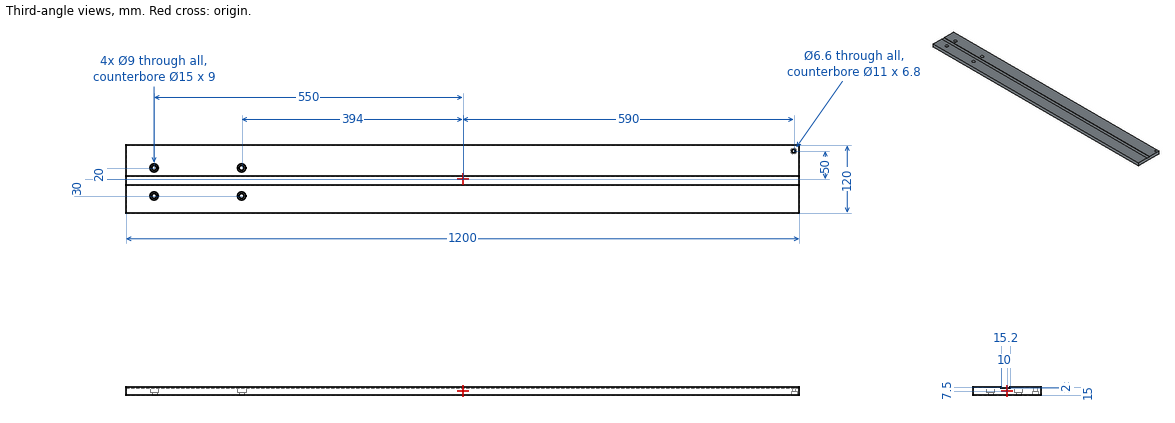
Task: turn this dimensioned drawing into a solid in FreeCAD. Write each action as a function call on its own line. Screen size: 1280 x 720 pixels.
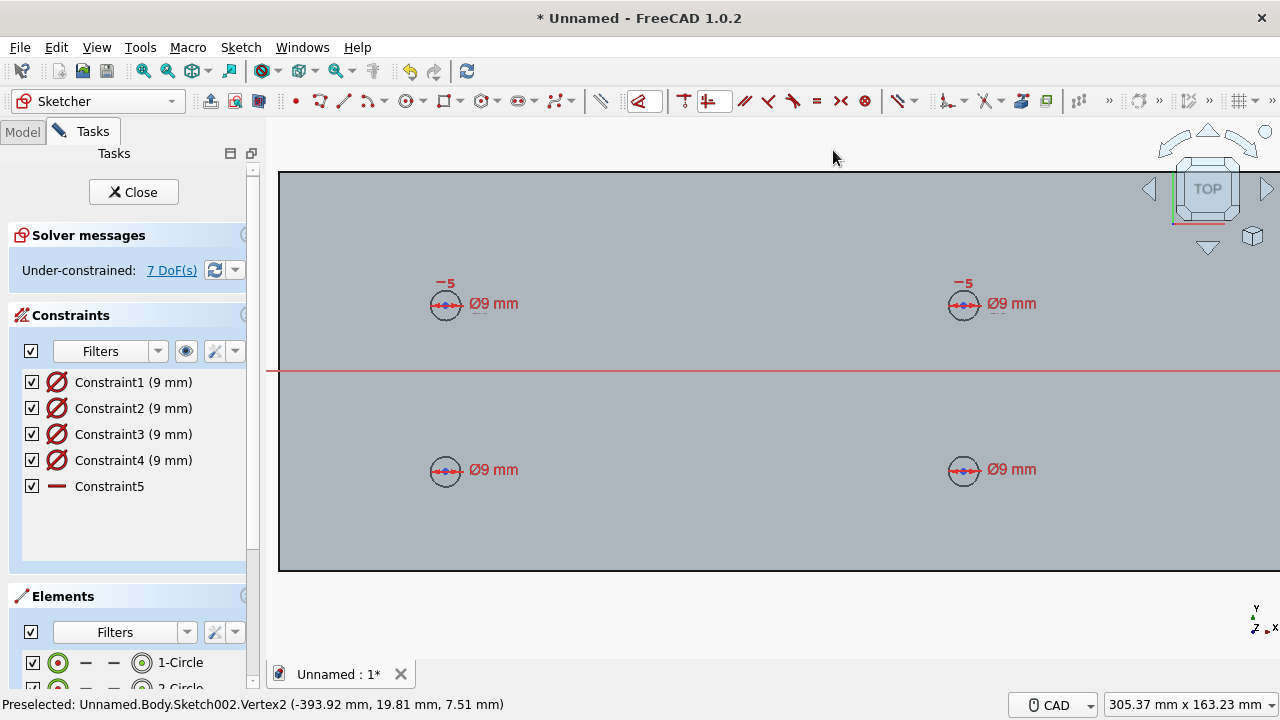
click(964, 306)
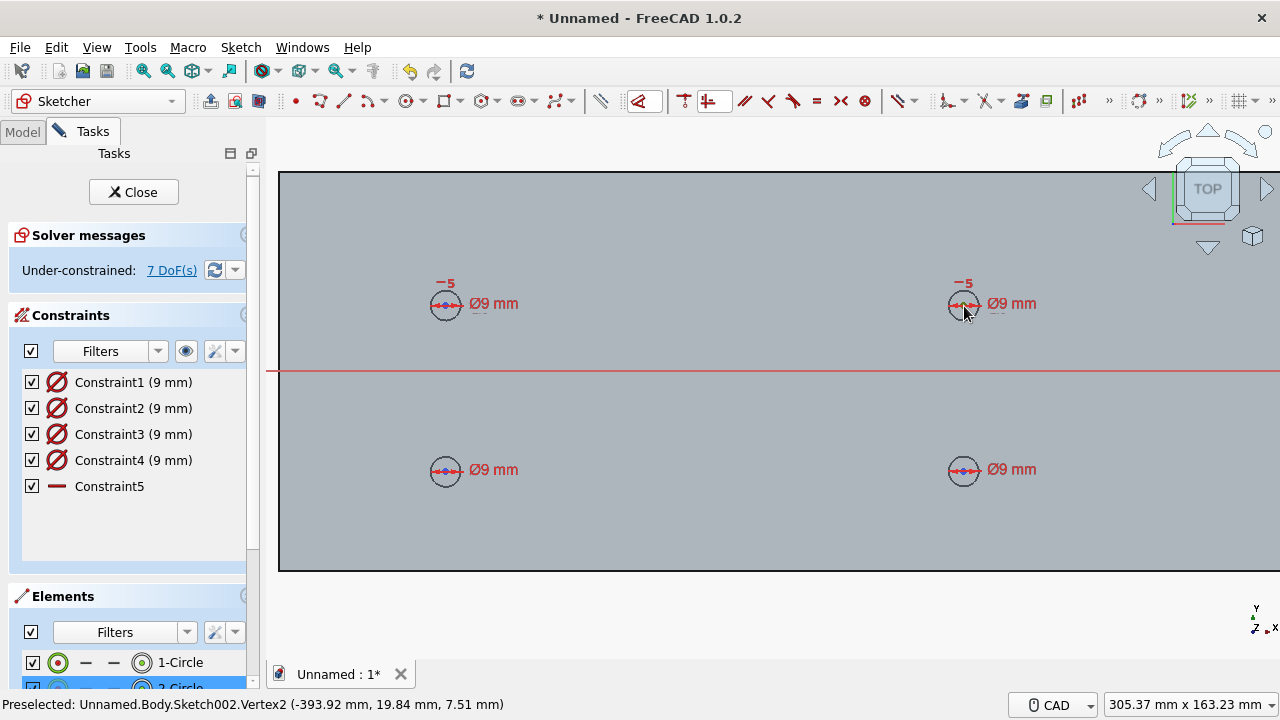
click(964, 471)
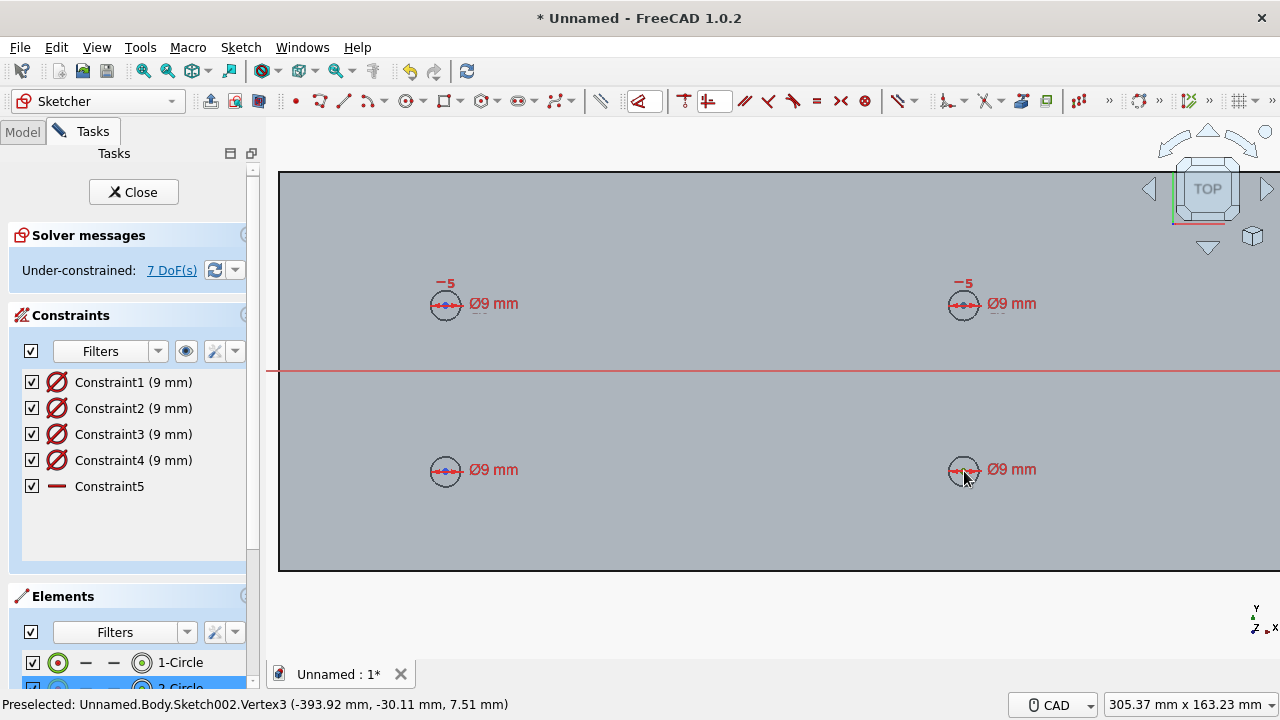
click(726, 102)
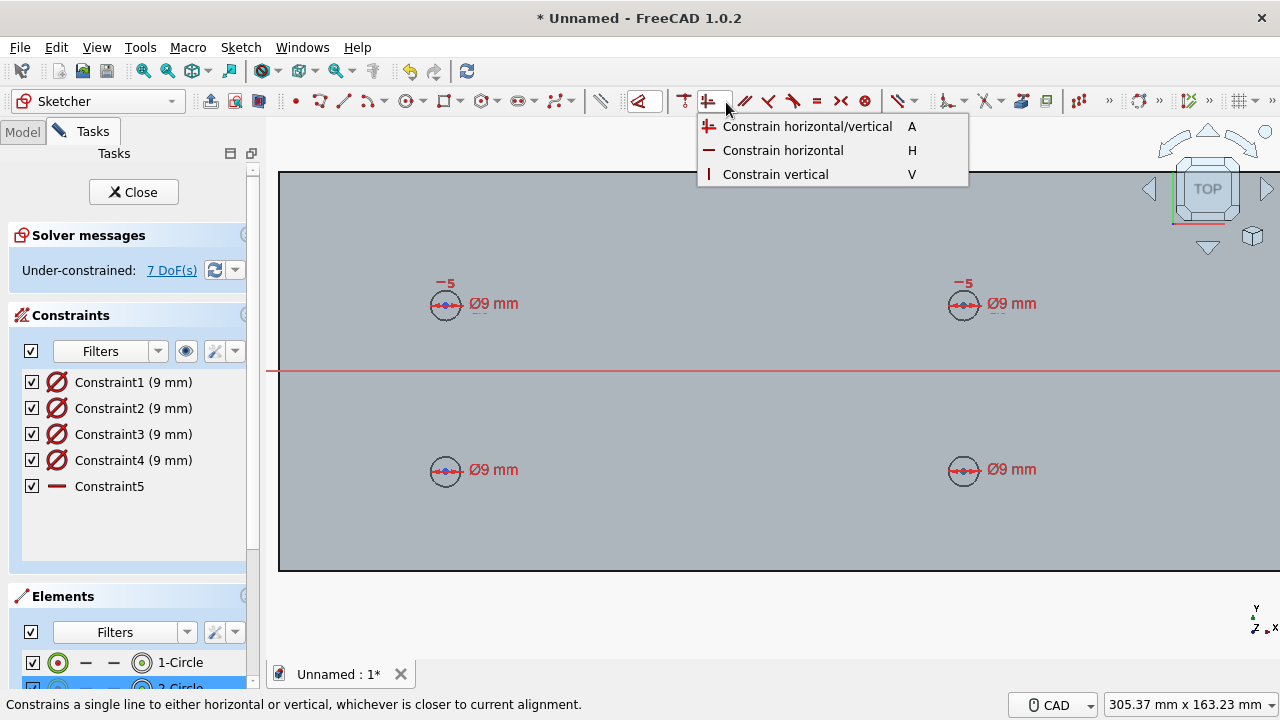
click(833, 174)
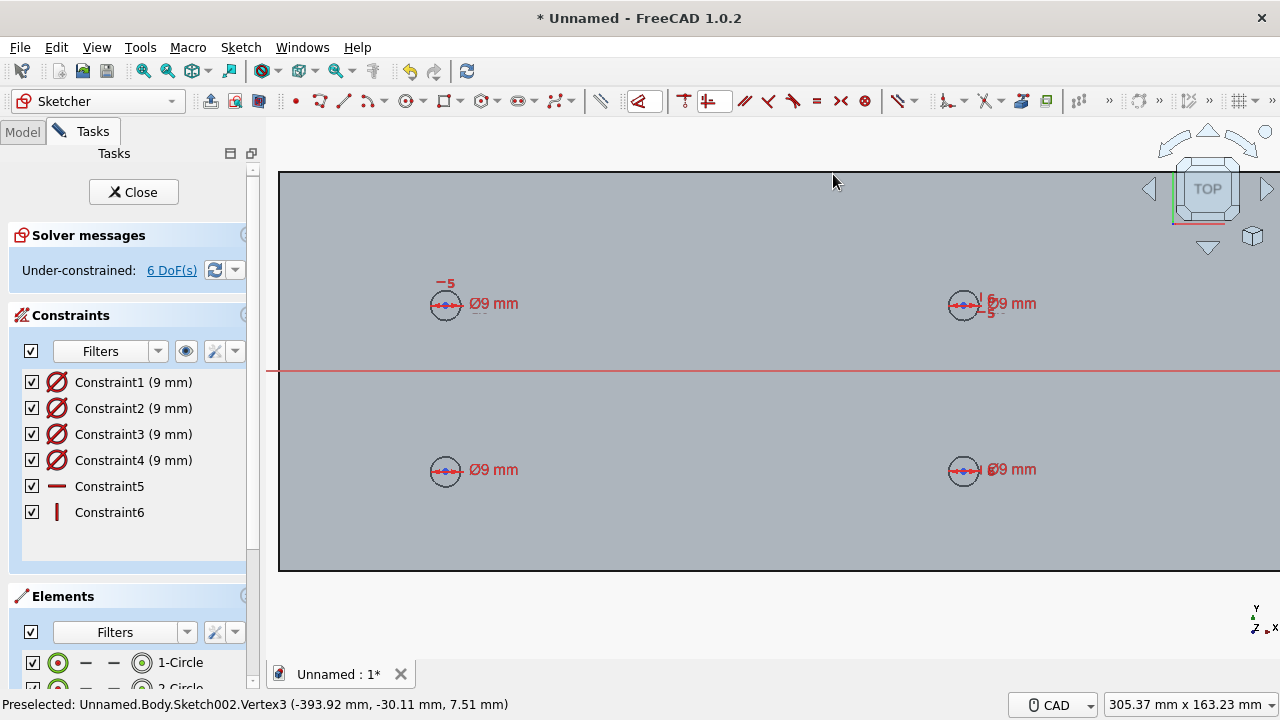
click(446, 306)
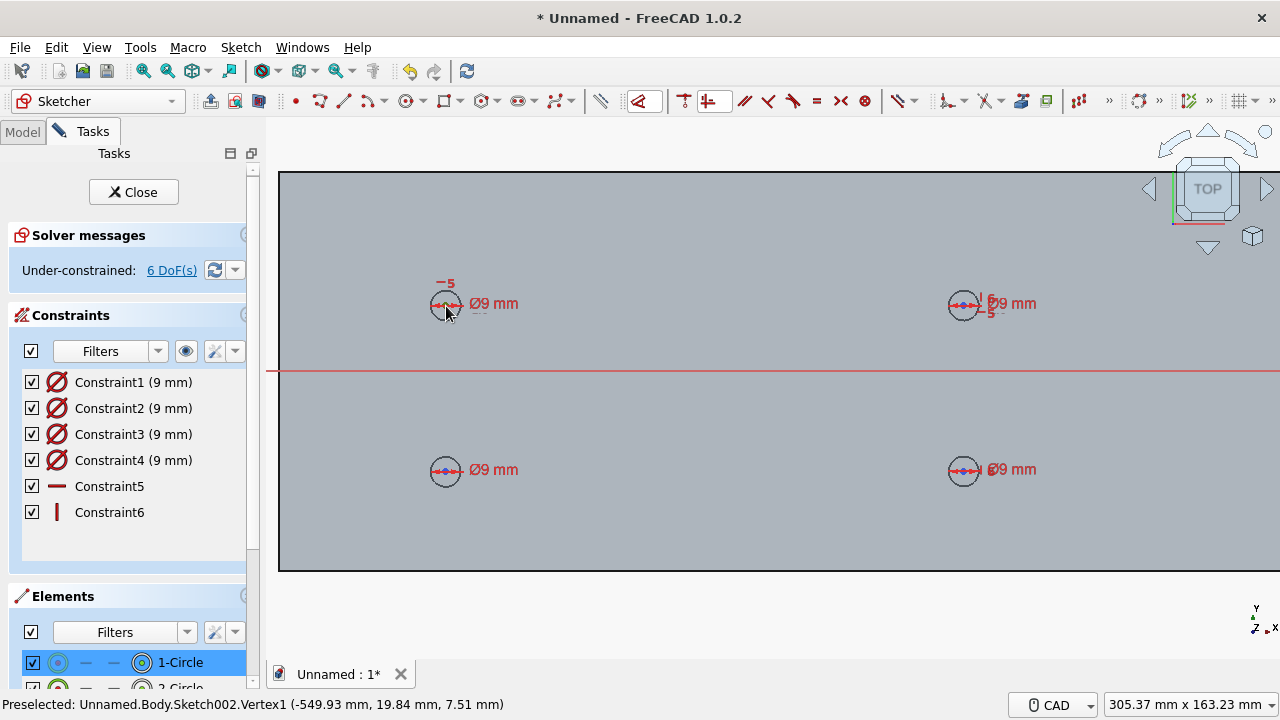
click(446, 472)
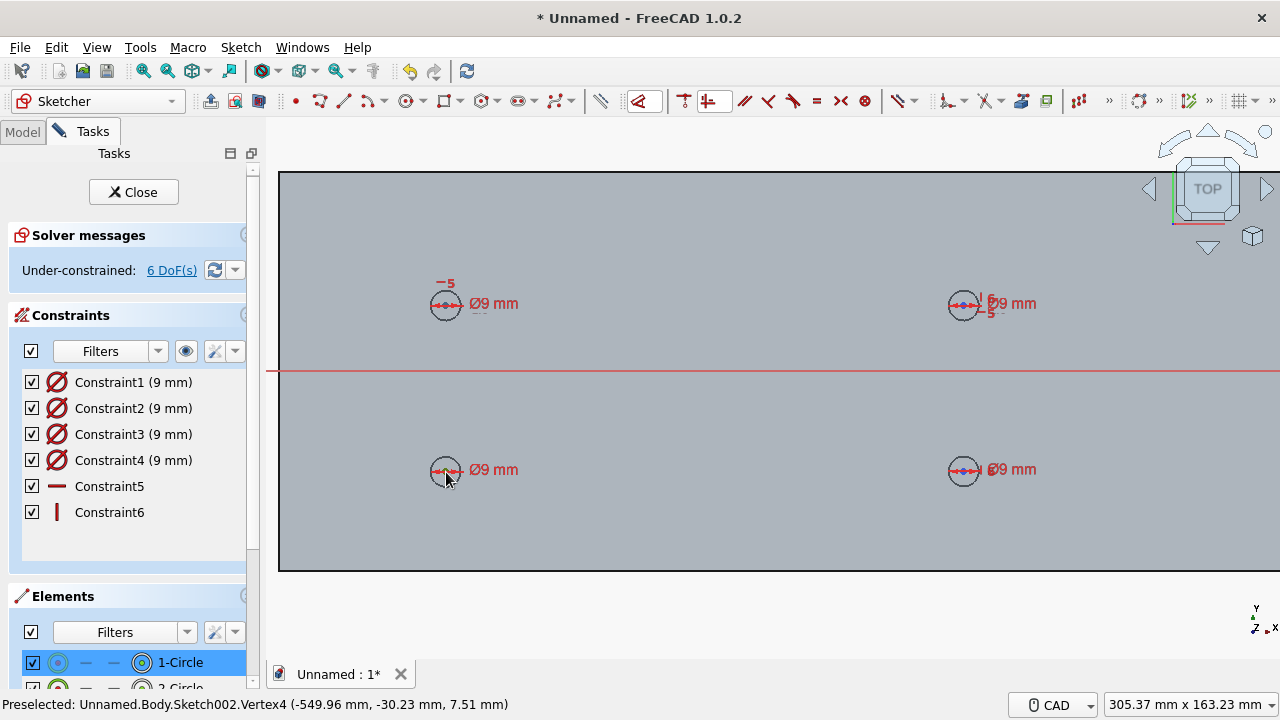
click(726, 102)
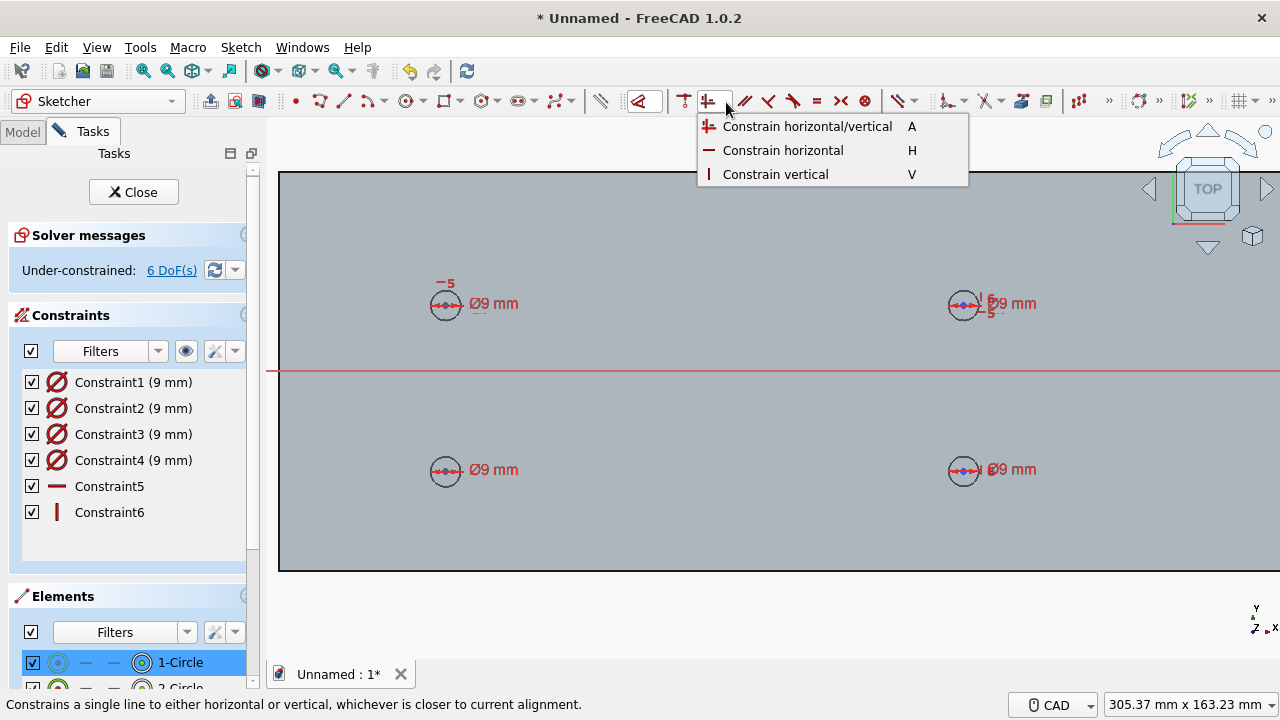
click(833, 174)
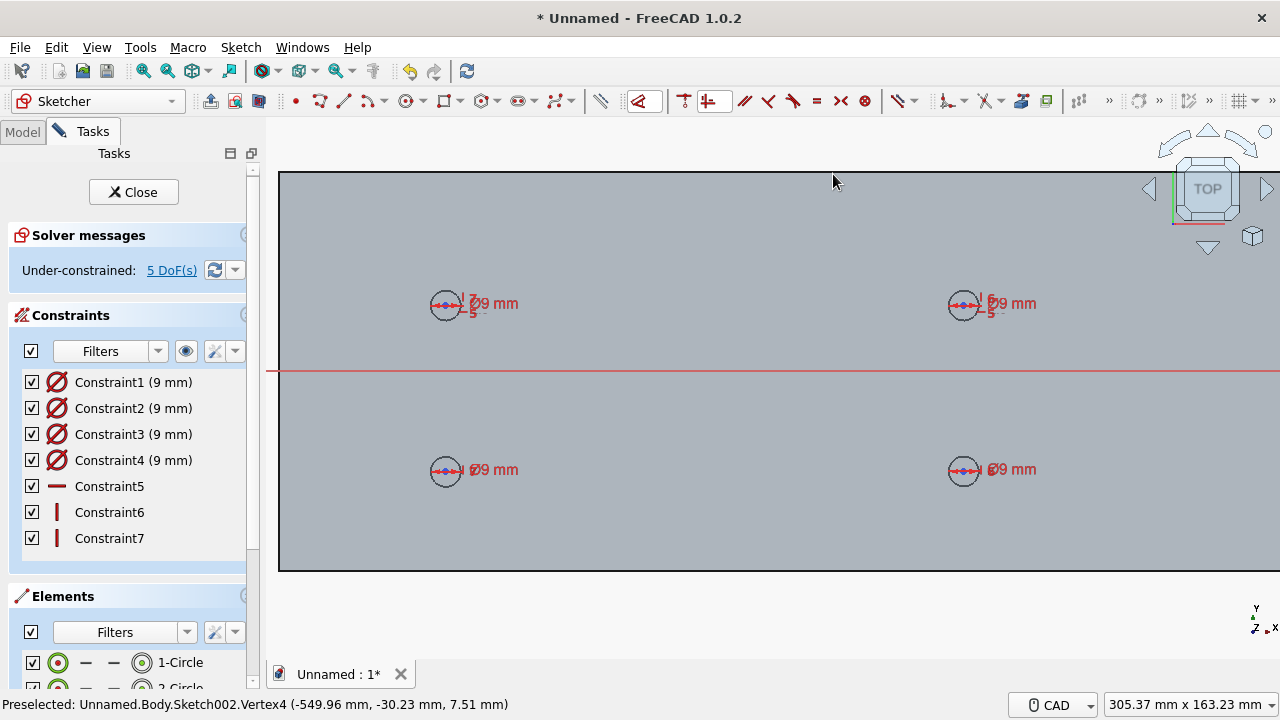
click(964, 471)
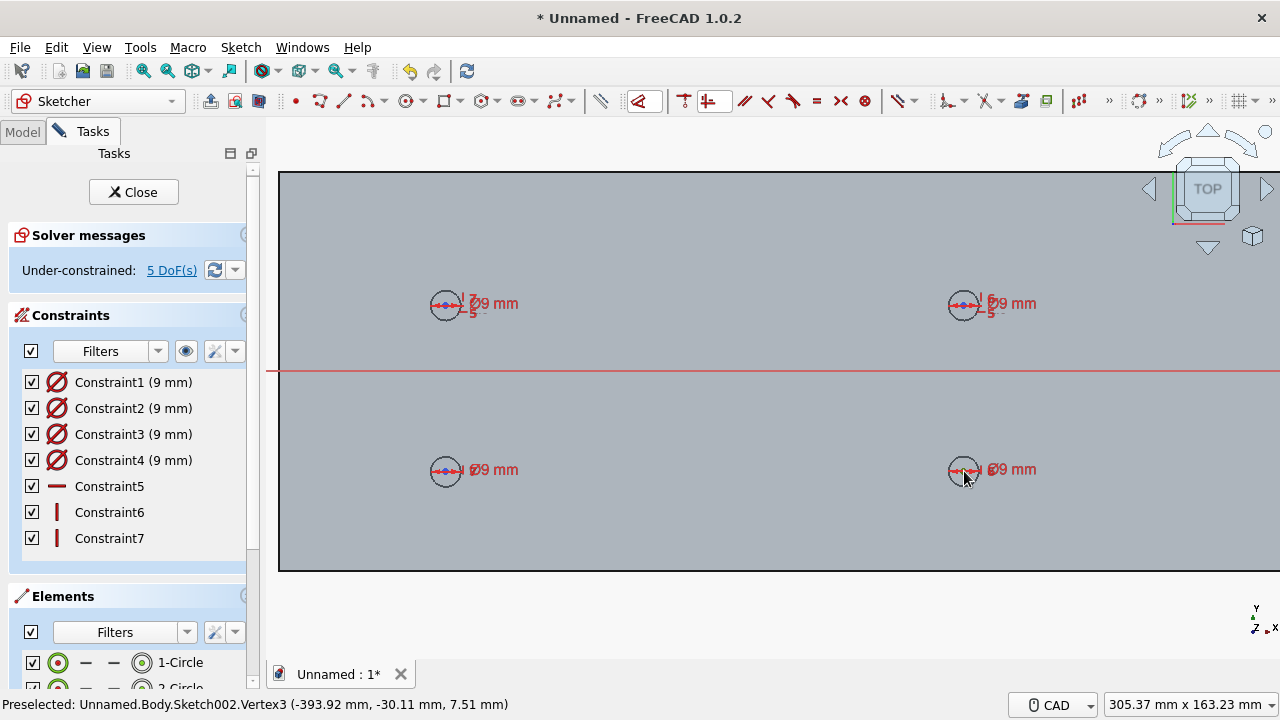
click(446, 472)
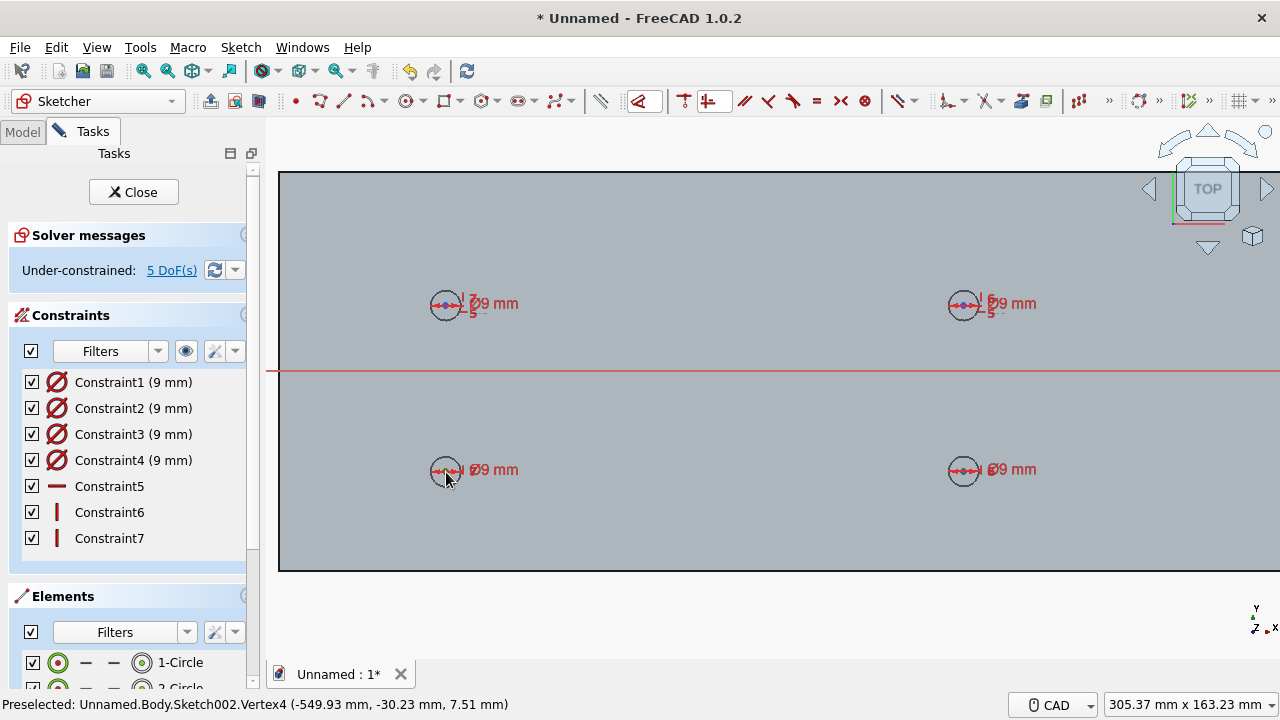
click(726, 102)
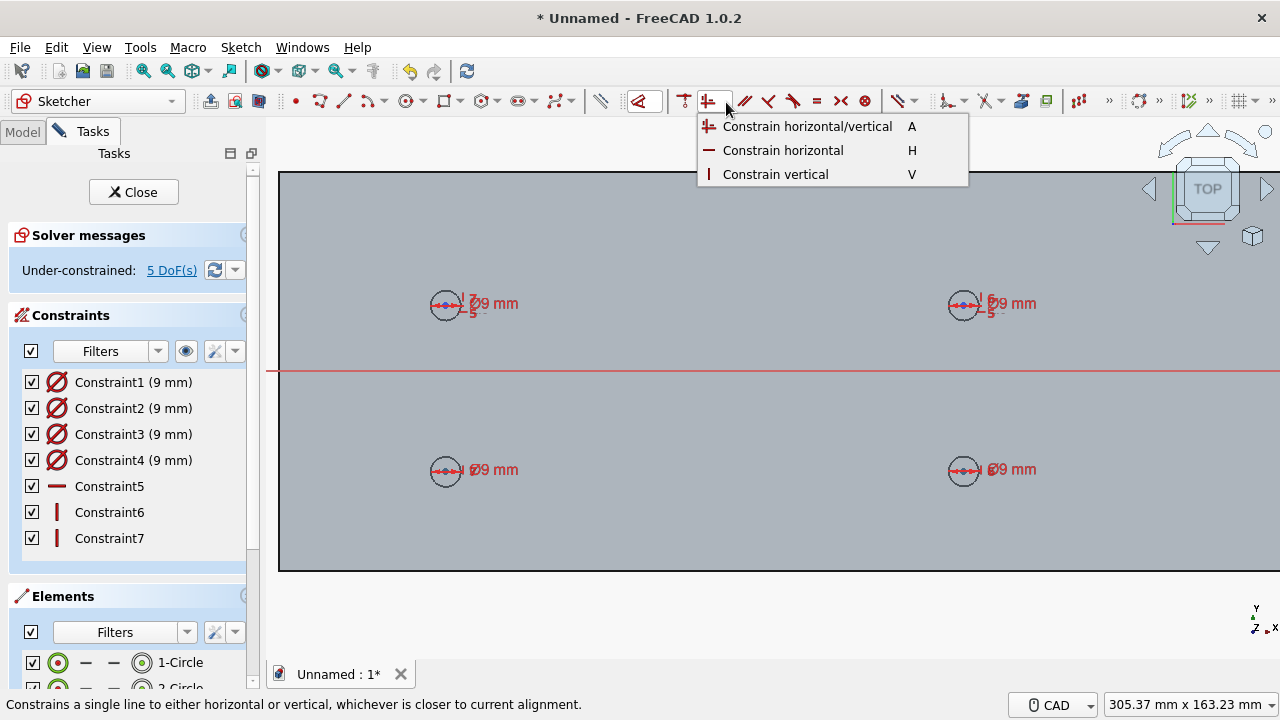
click(833, 150)